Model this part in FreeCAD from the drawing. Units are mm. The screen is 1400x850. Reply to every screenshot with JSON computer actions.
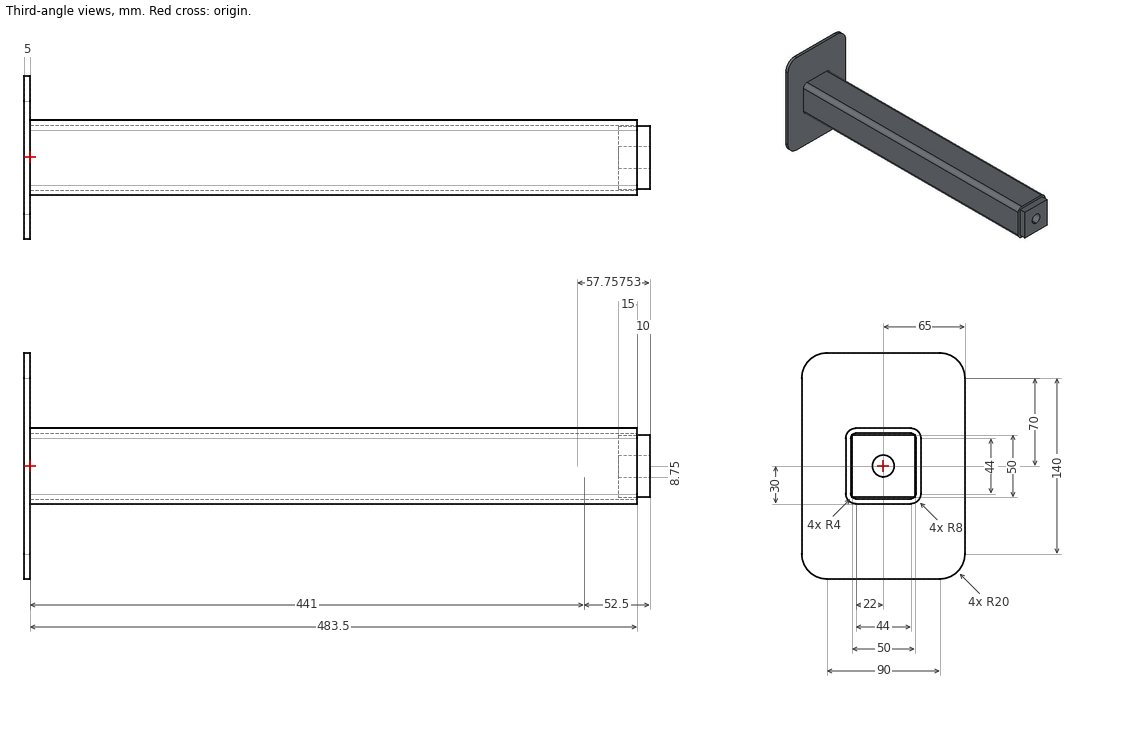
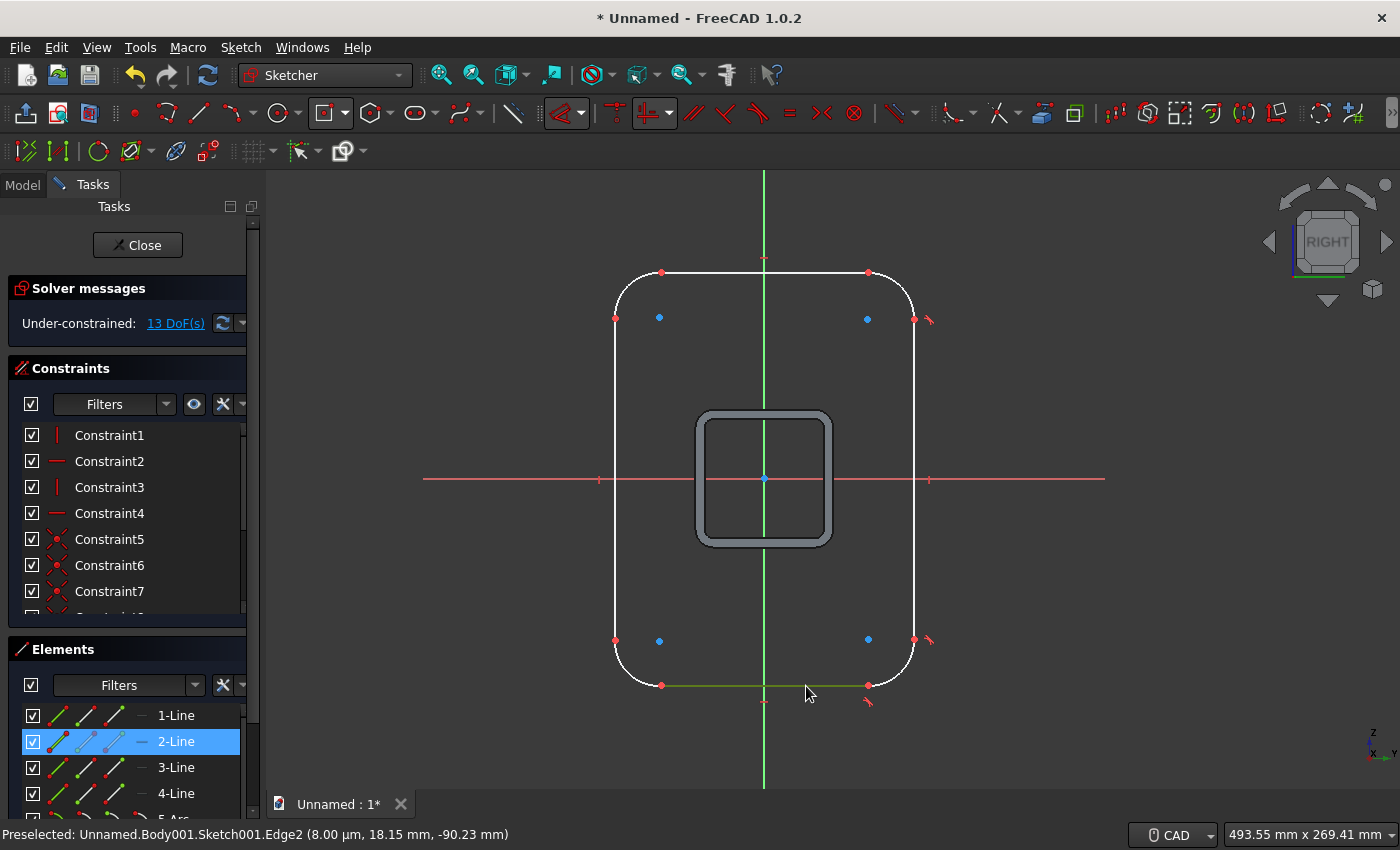
{"action": "left_click", "coordinate": [620, 662]}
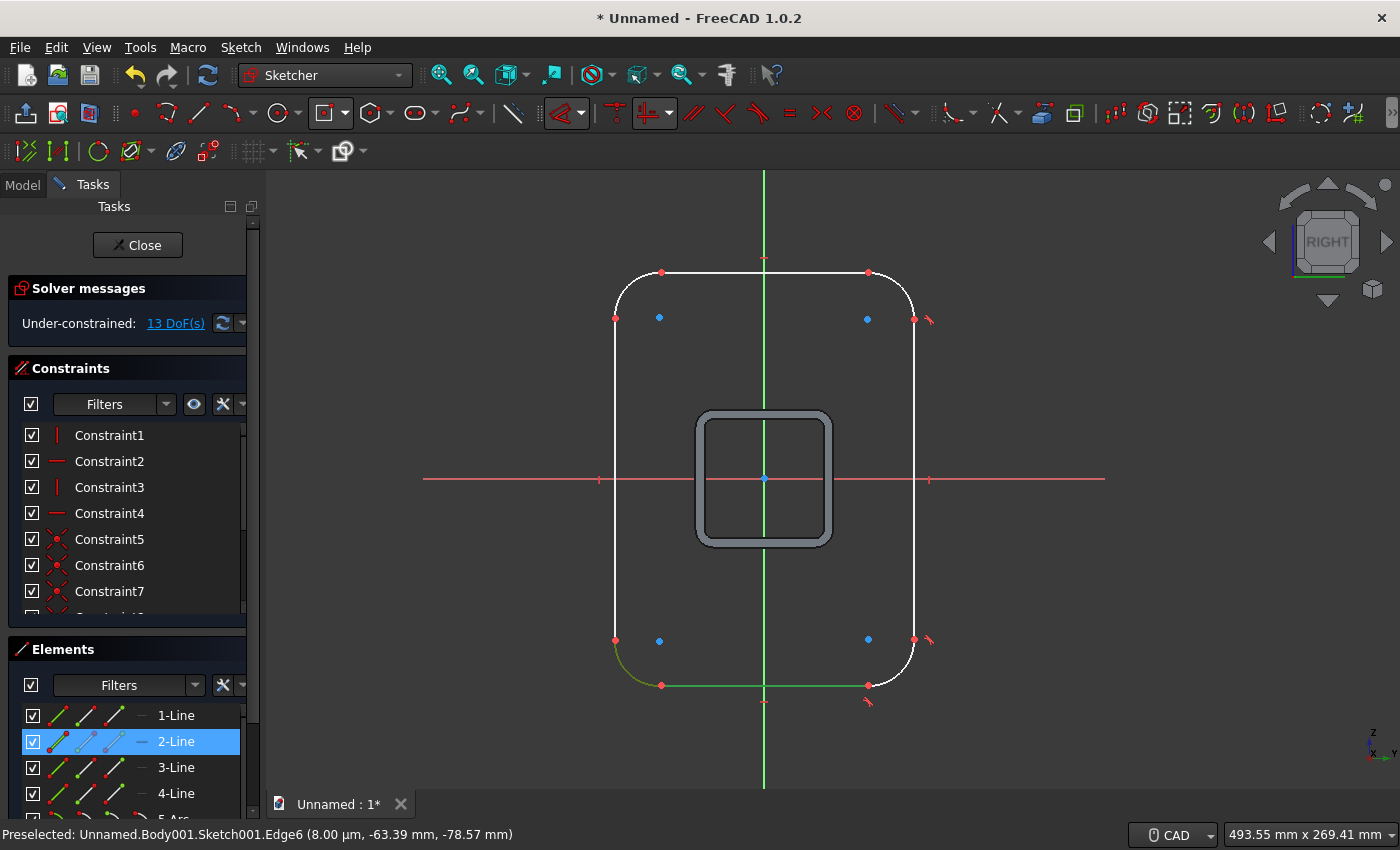
{"action": "left_click", "coordinate": [758, 114]}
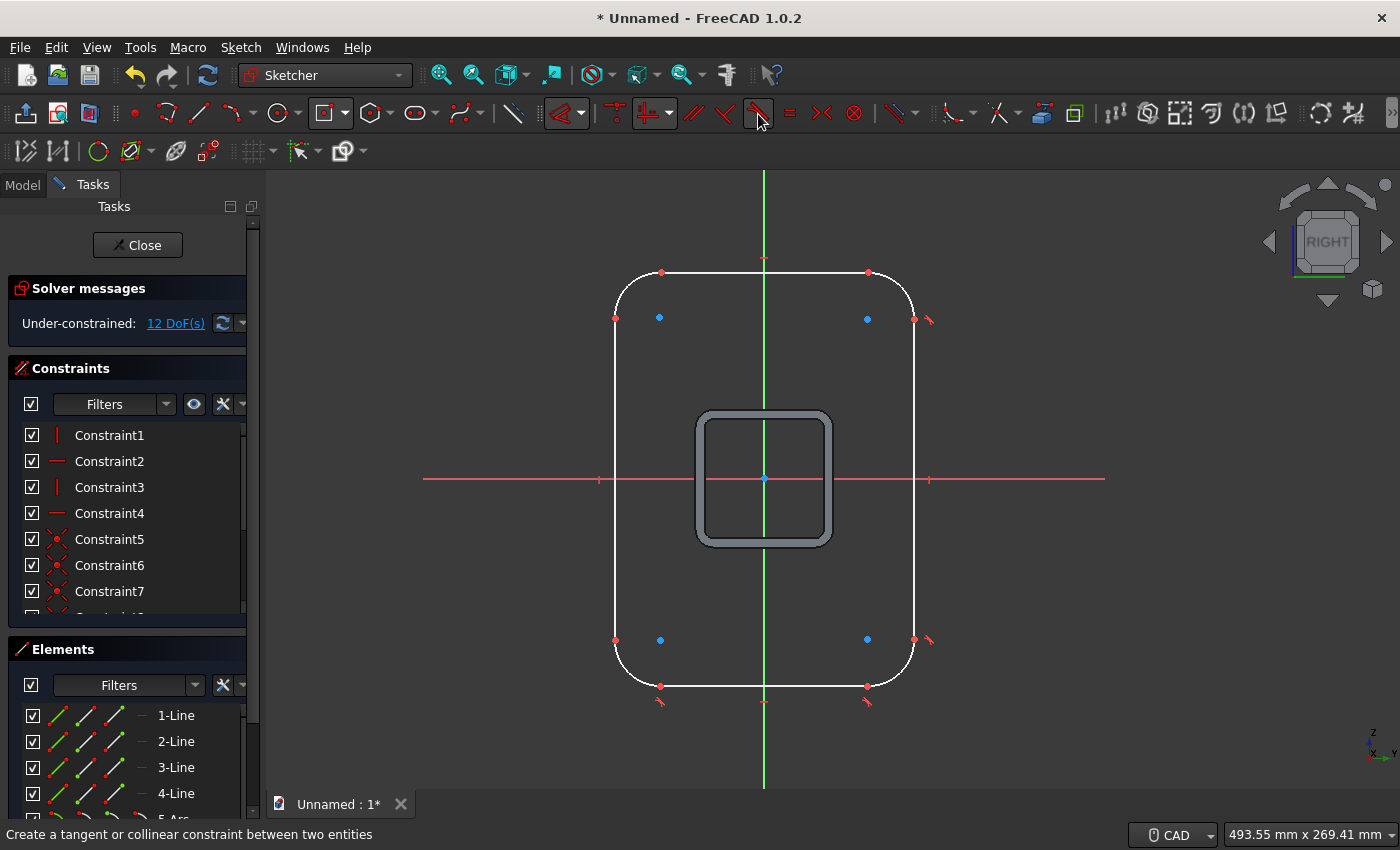
{"action": "left_click", "coordinate": [615, 544]}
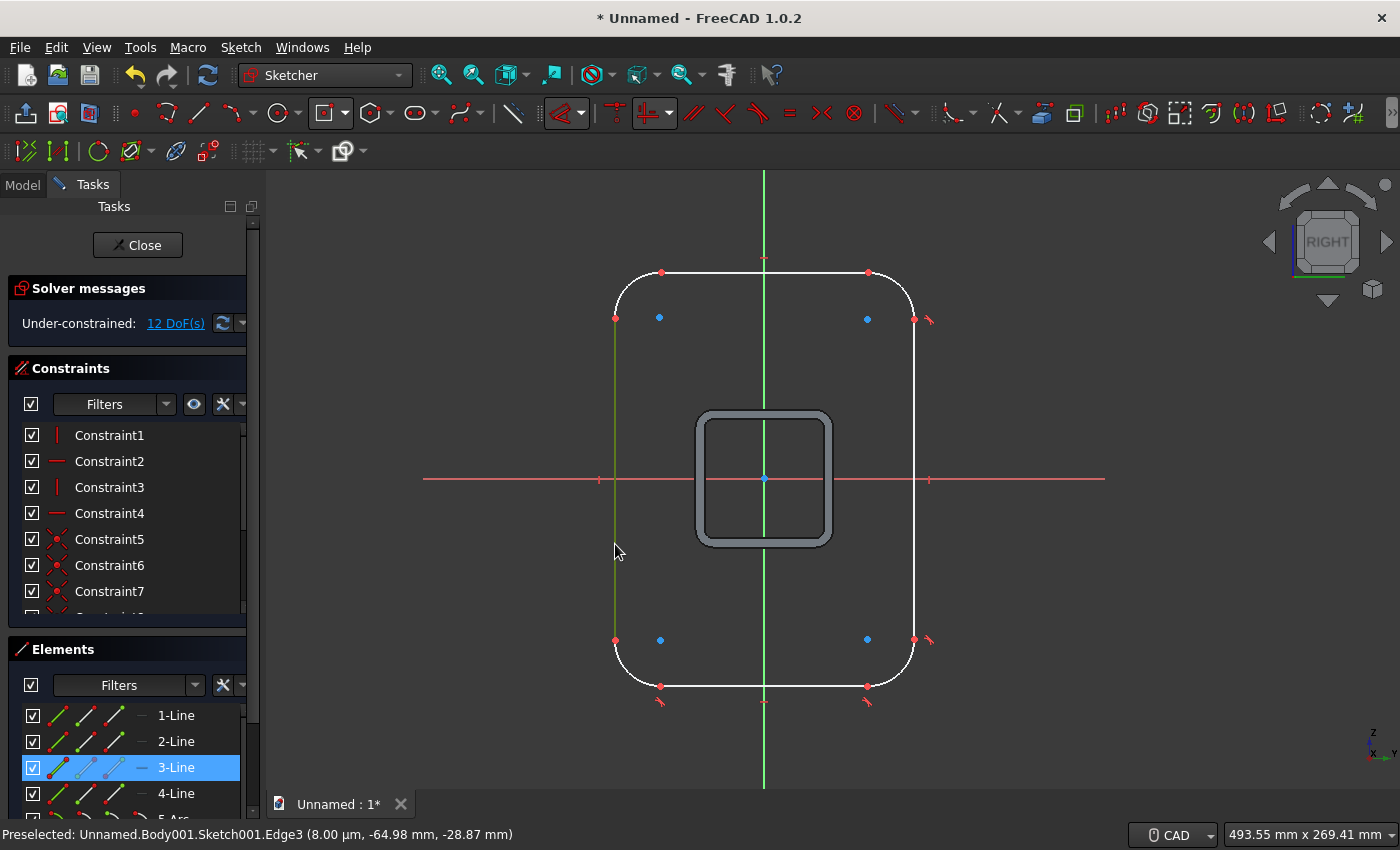
{"action": "left_click", "coordinate": [620, 662]}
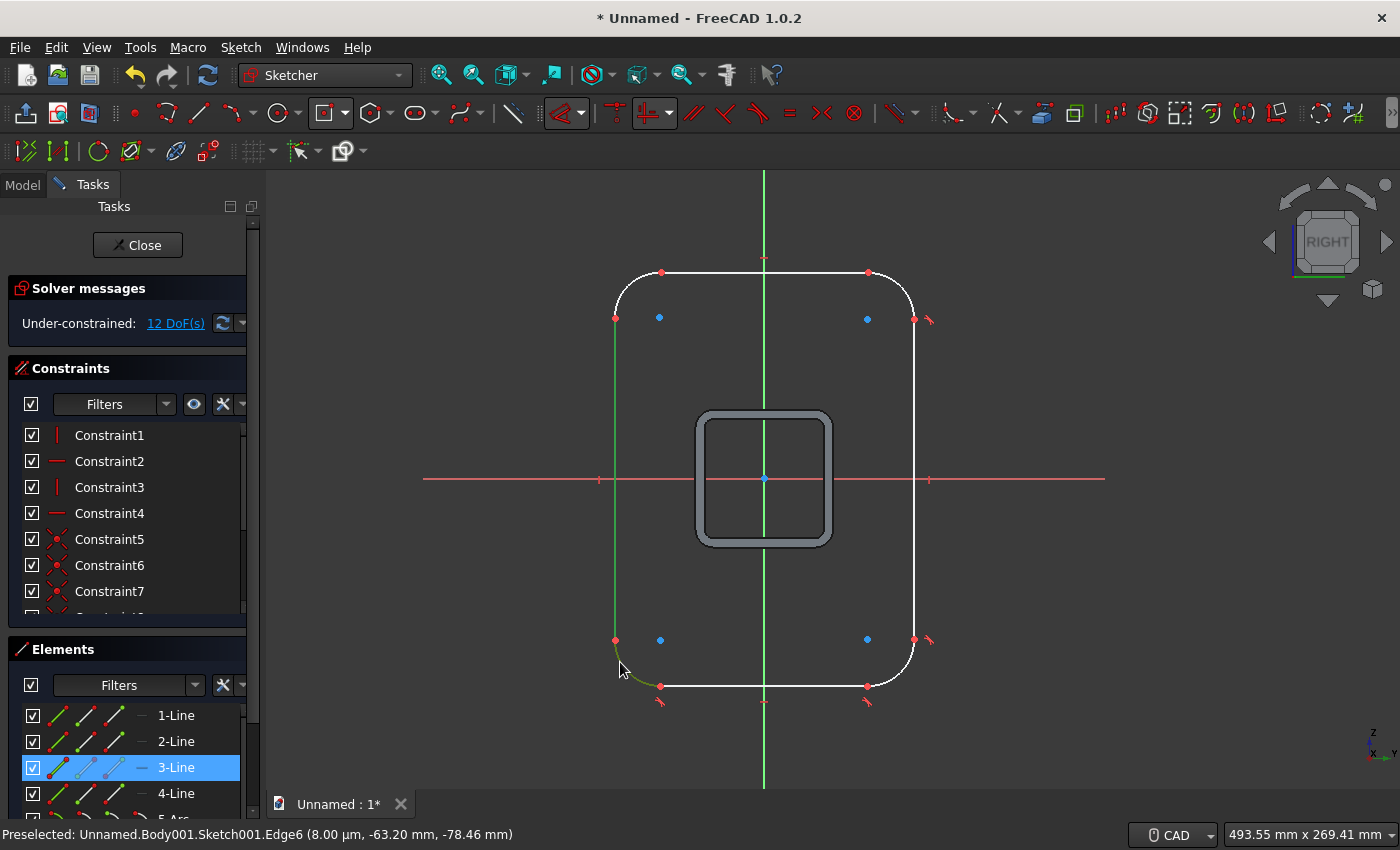
{"action": "key", "text": "t"}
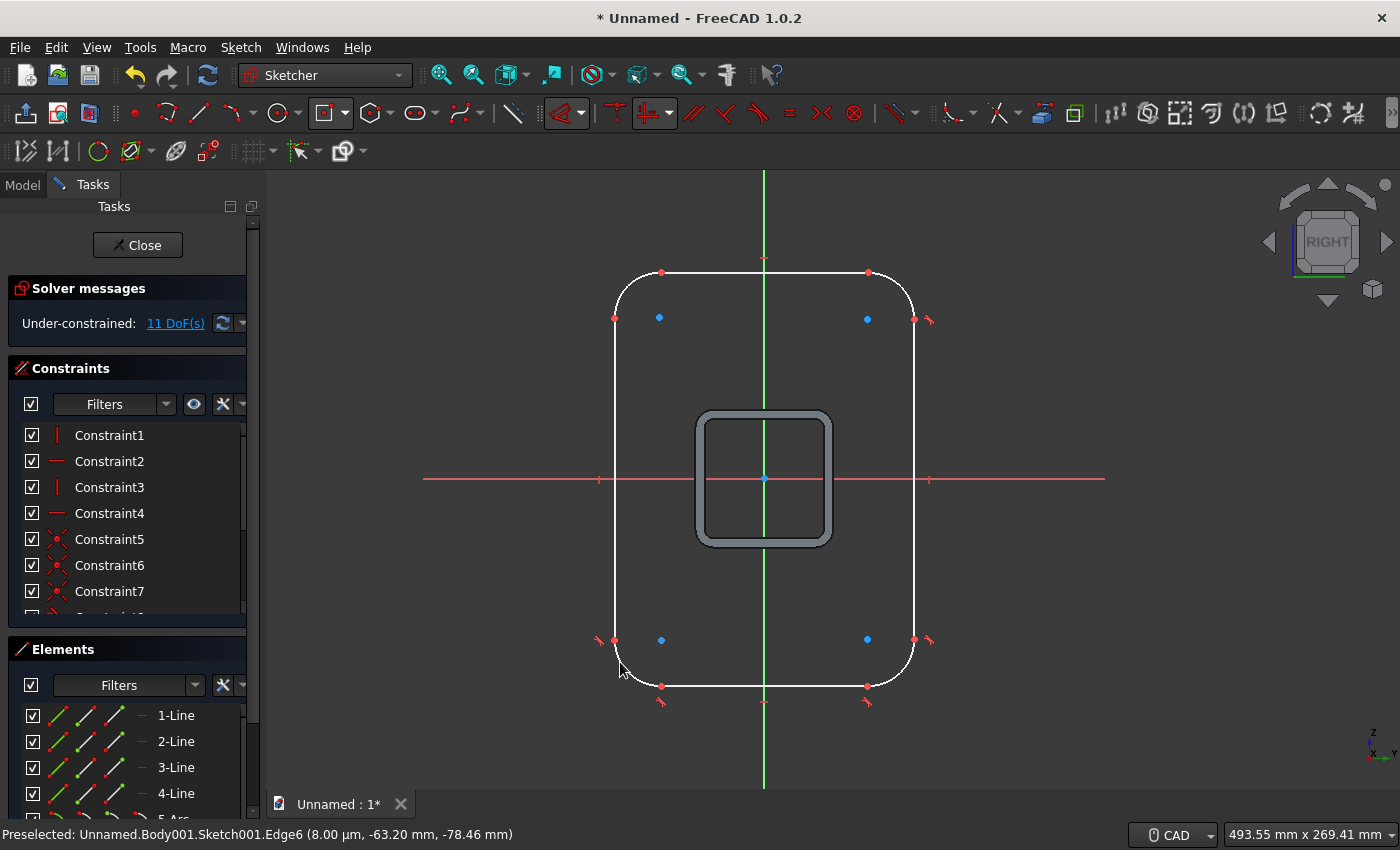
{"action": "left_click", "coordinate": [615, 544]}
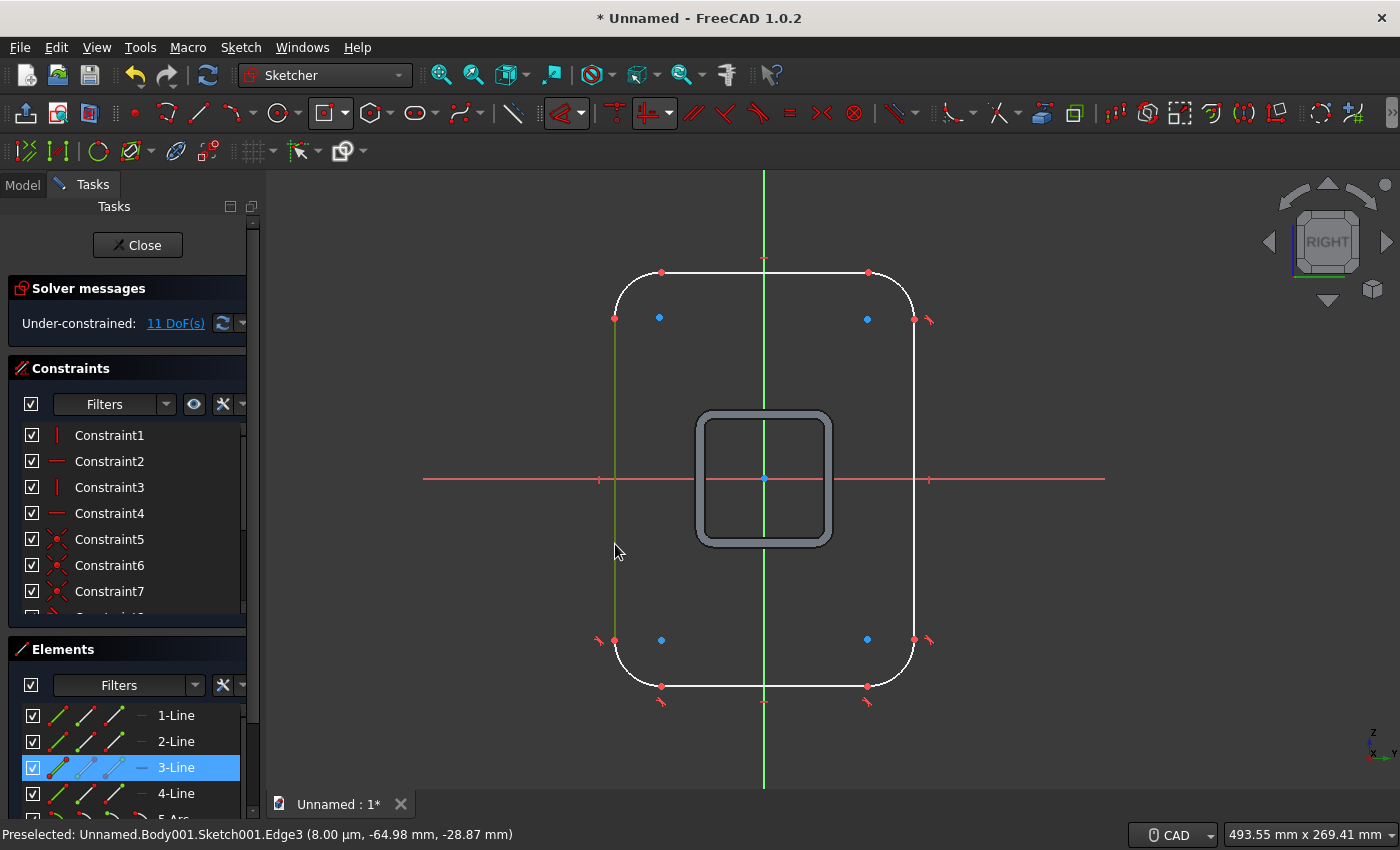
{"action": "left_click", "coordinate": [640, 277]}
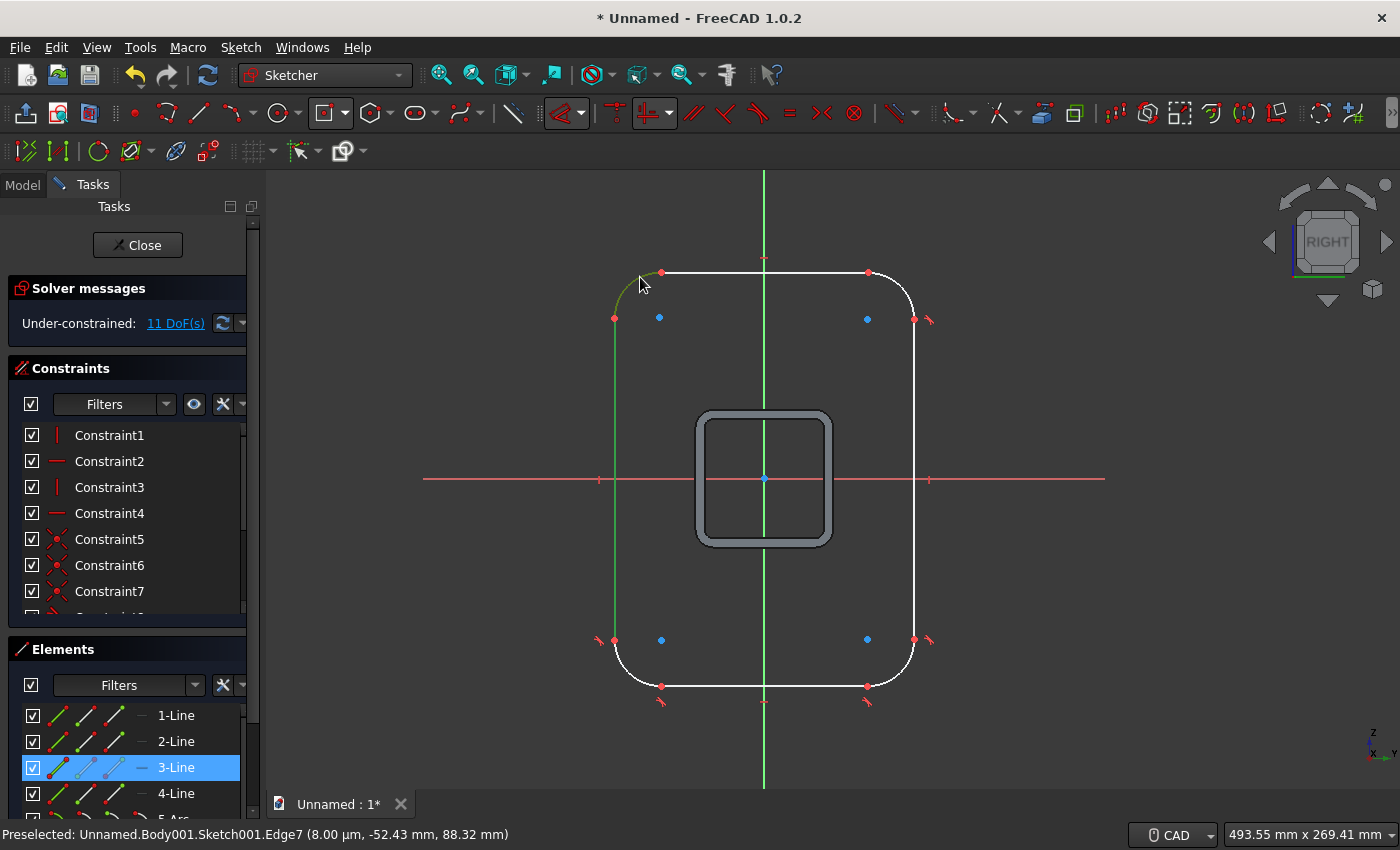
{"action": "left_click", "coordinate": [758, 114]}